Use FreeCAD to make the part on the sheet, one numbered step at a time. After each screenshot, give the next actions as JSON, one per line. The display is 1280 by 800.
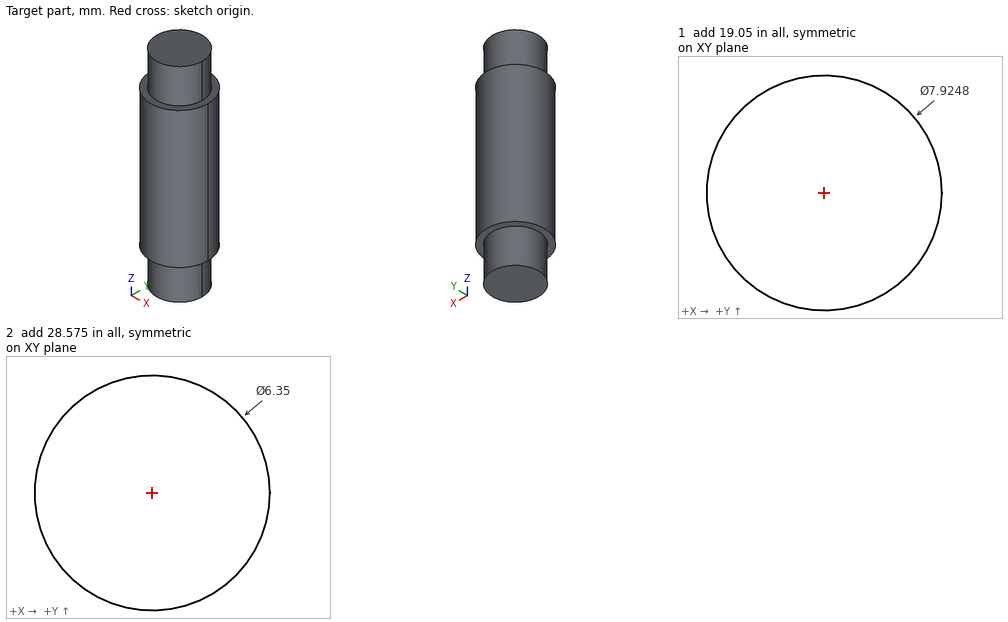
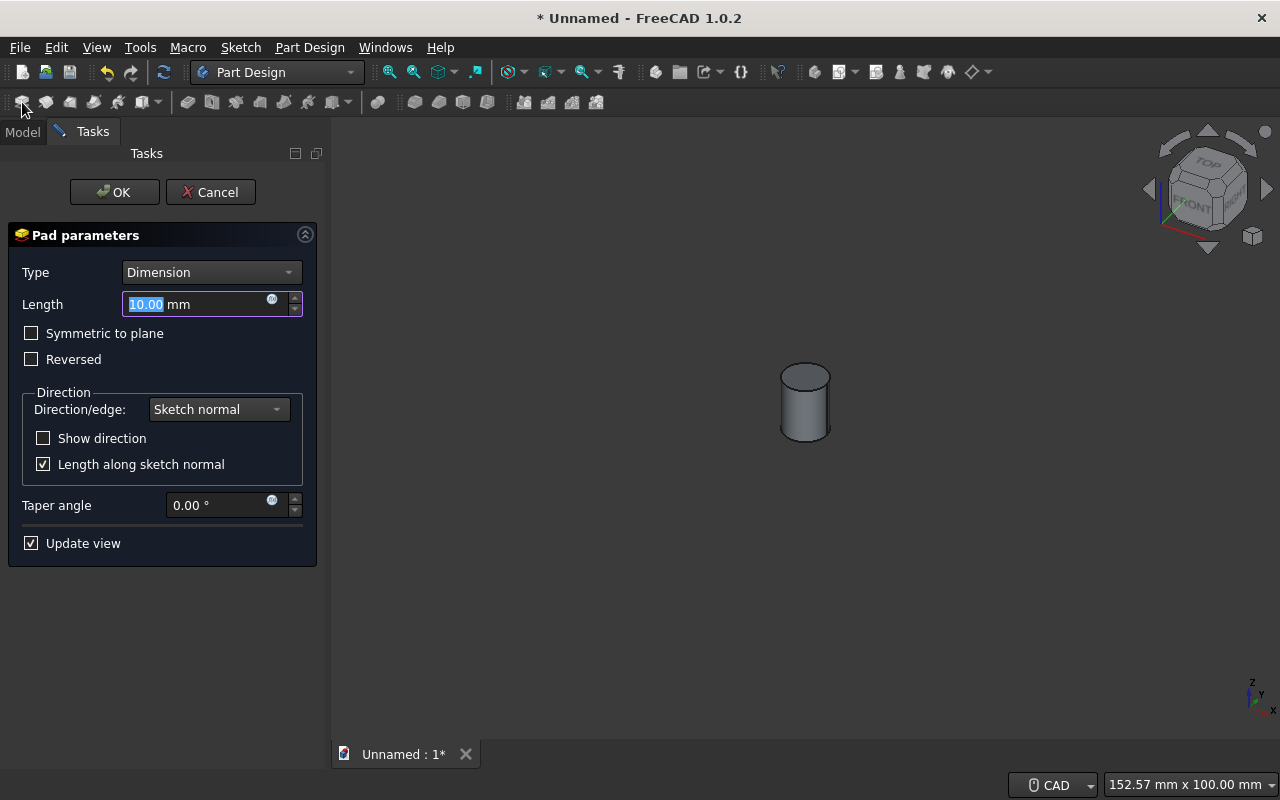
{"action": "type", "text": "19.05"}
{"action": "key", "text": "Tab"}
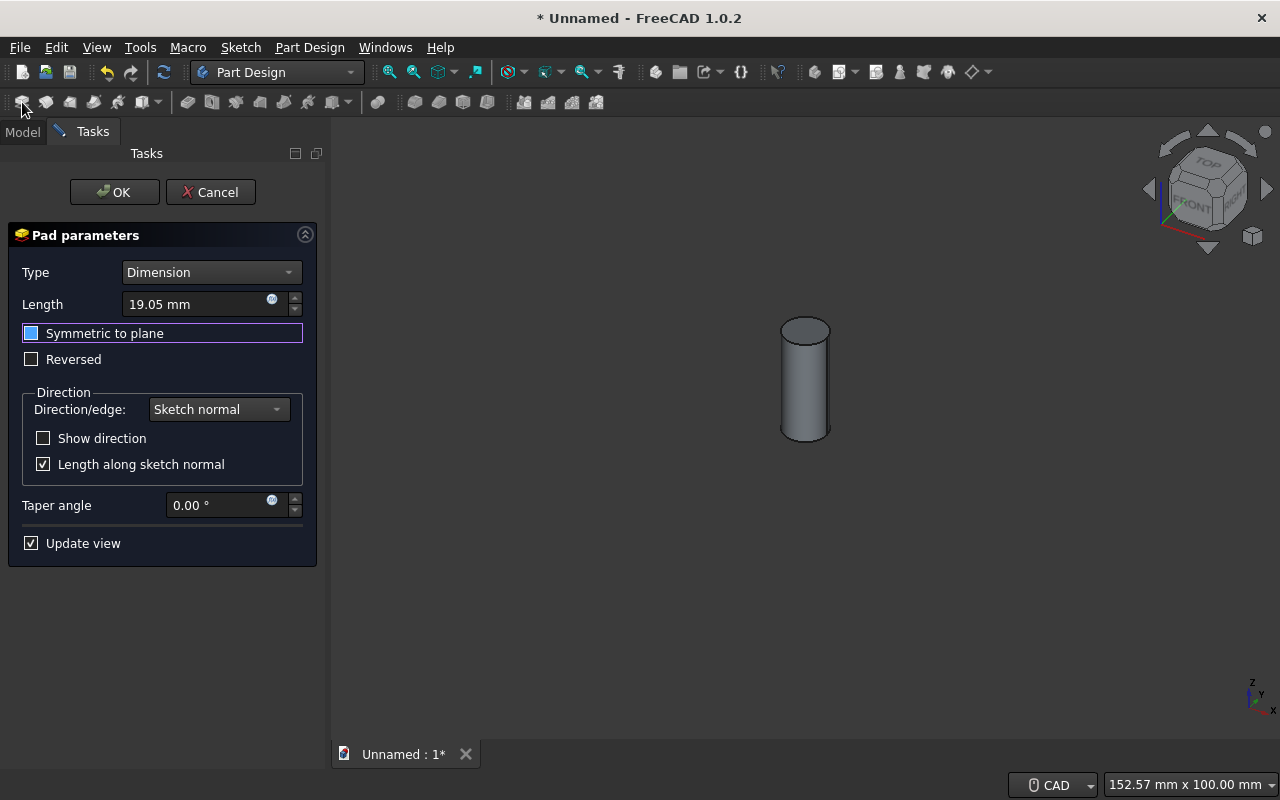
{"action": "left_click", "coordinate": [30, 333]}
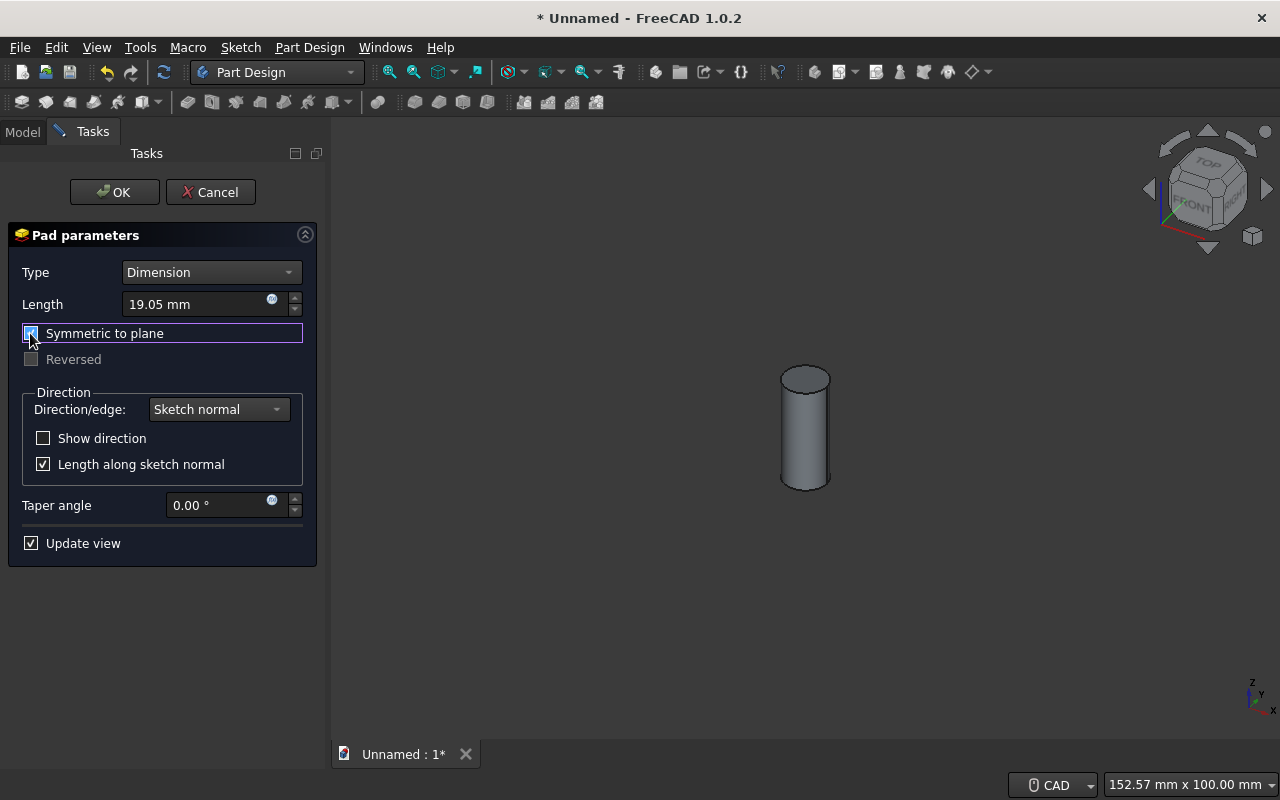
{"action": "left_click", "coordinate": [115, 192]}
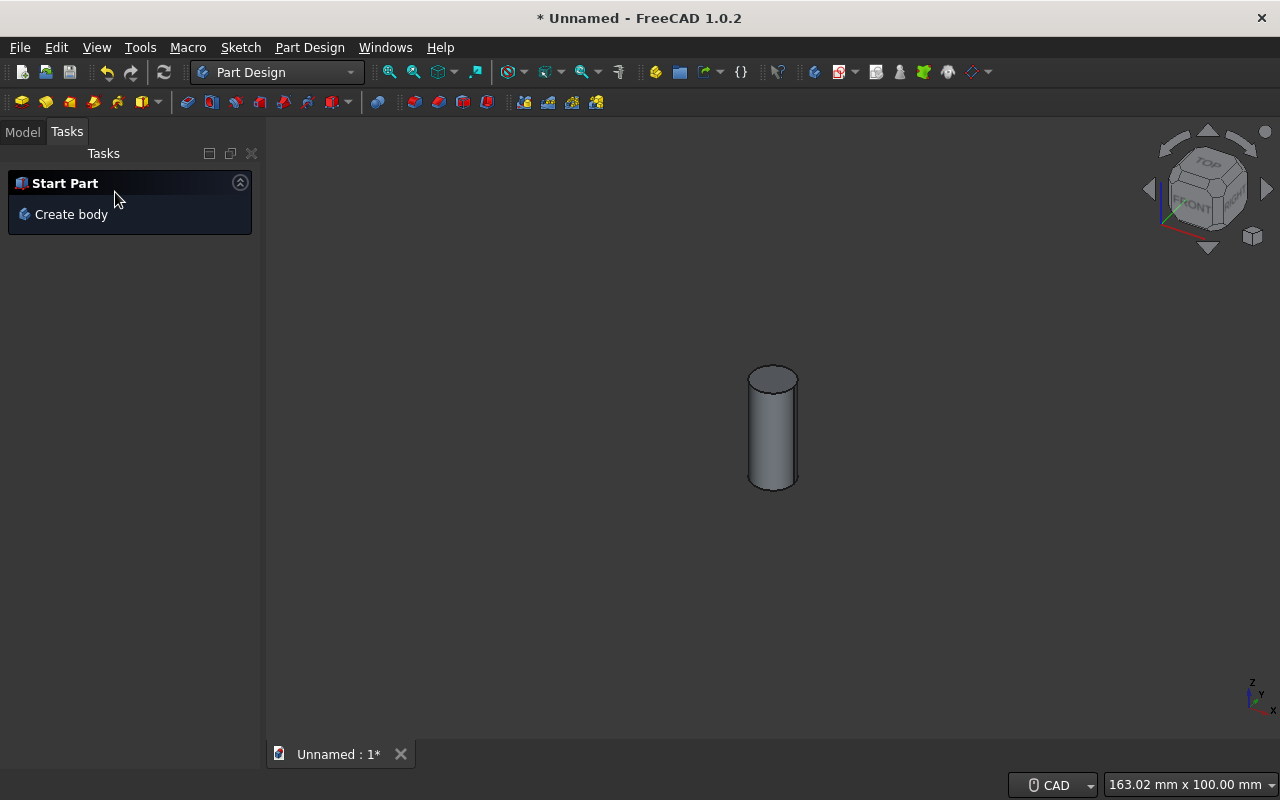
{"action": "key", "text": "v f"}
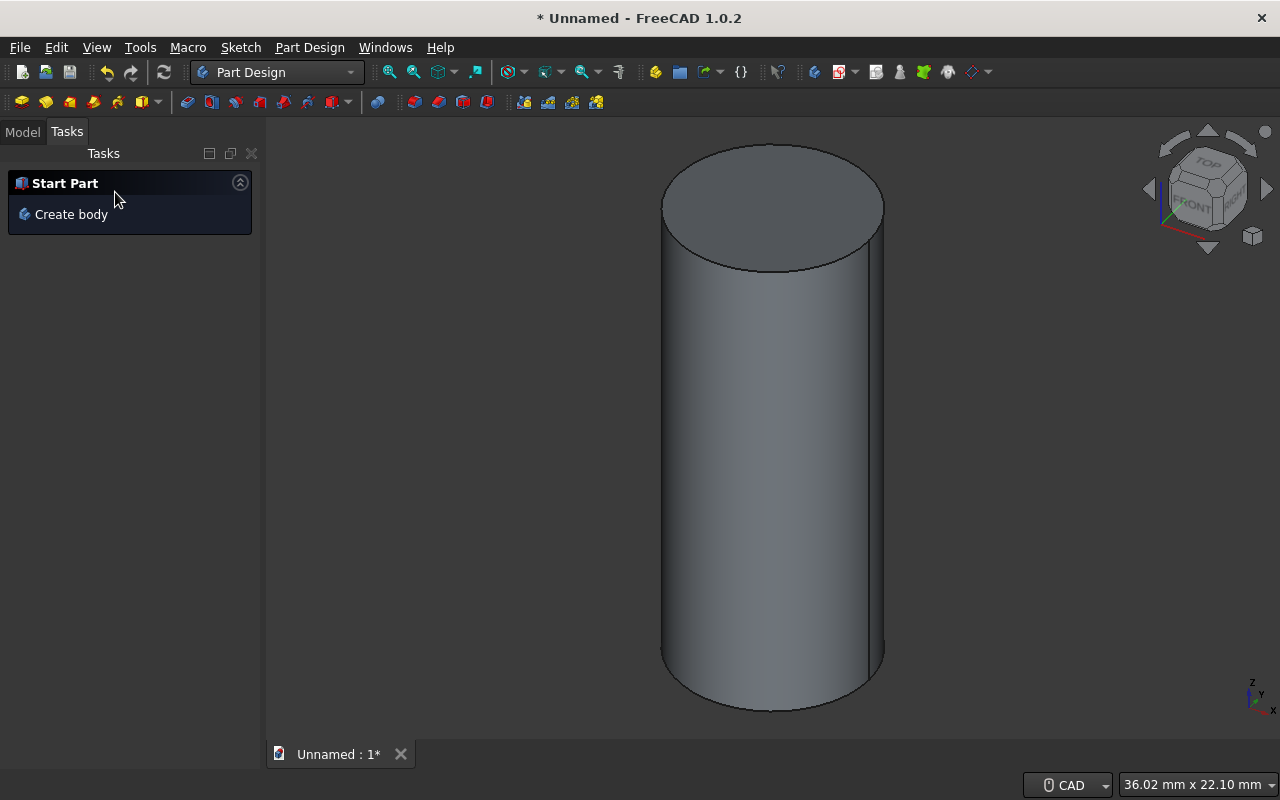
{"action": "left_click", "coordinate": [840, 72]}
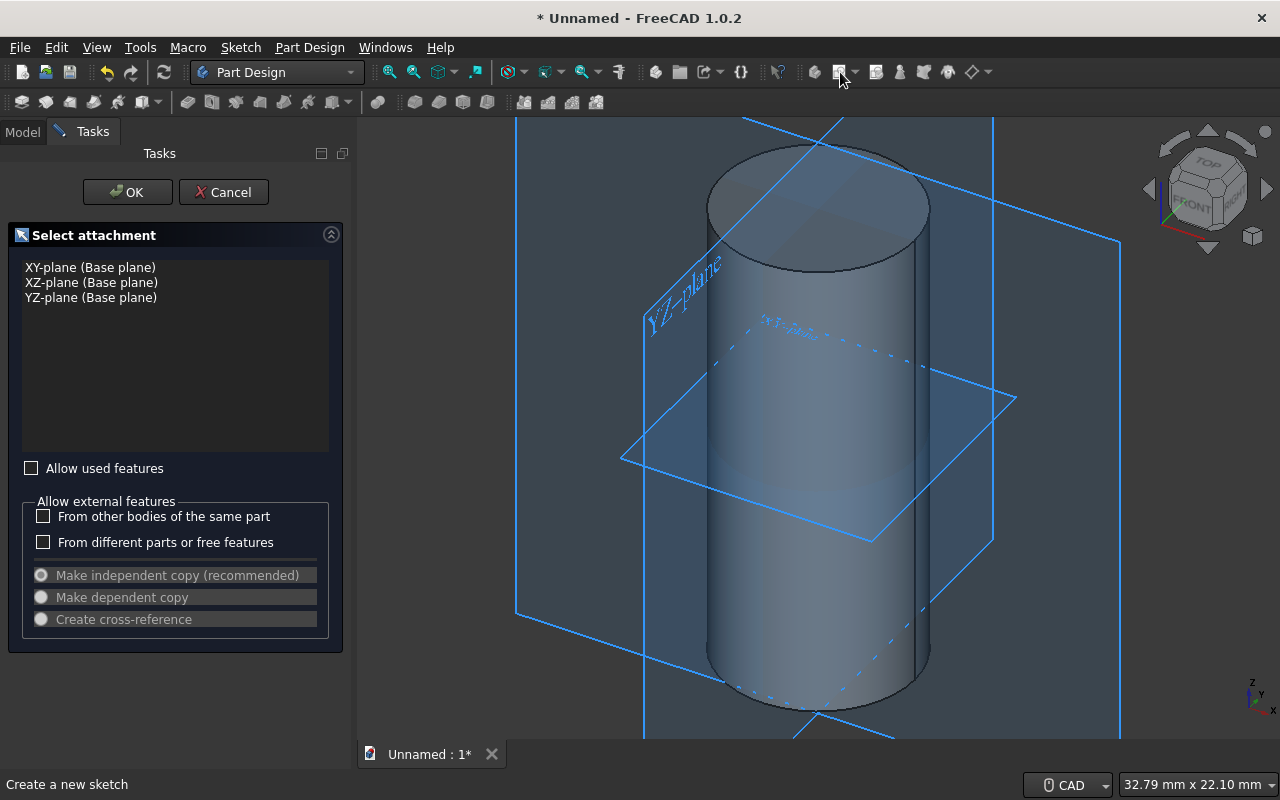
{"action": "left_click", "coordinate": [82, 268]}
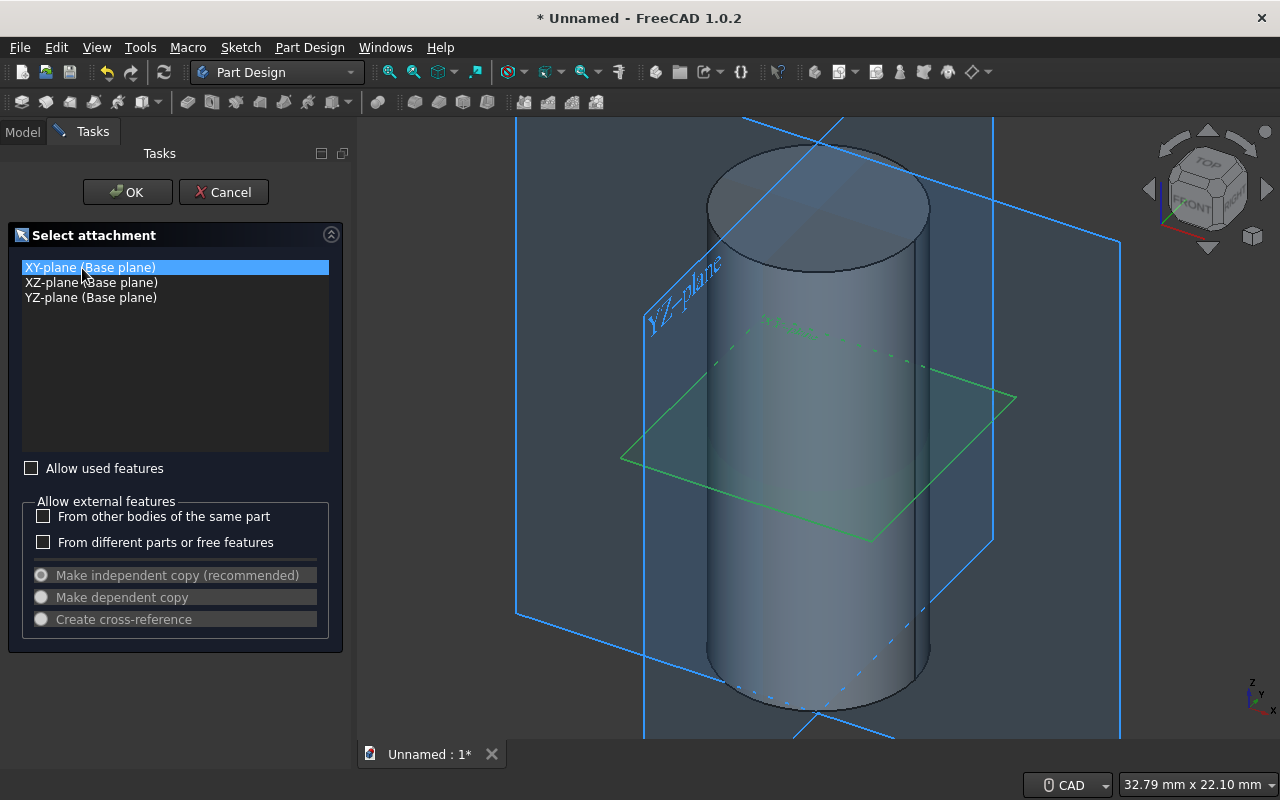
{"action": "left_click", "coordinate": [128, 192]}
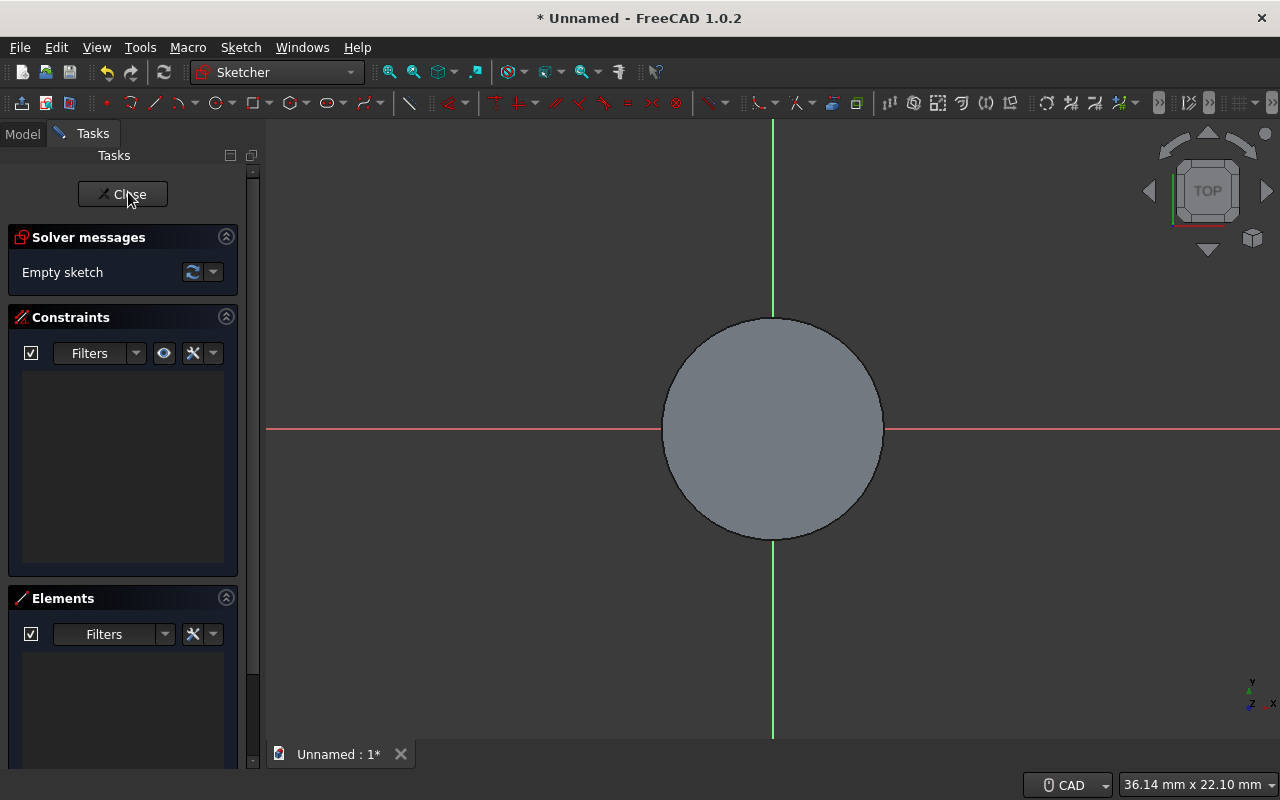
{"action": "left_click", "coordinate": [70, 104]}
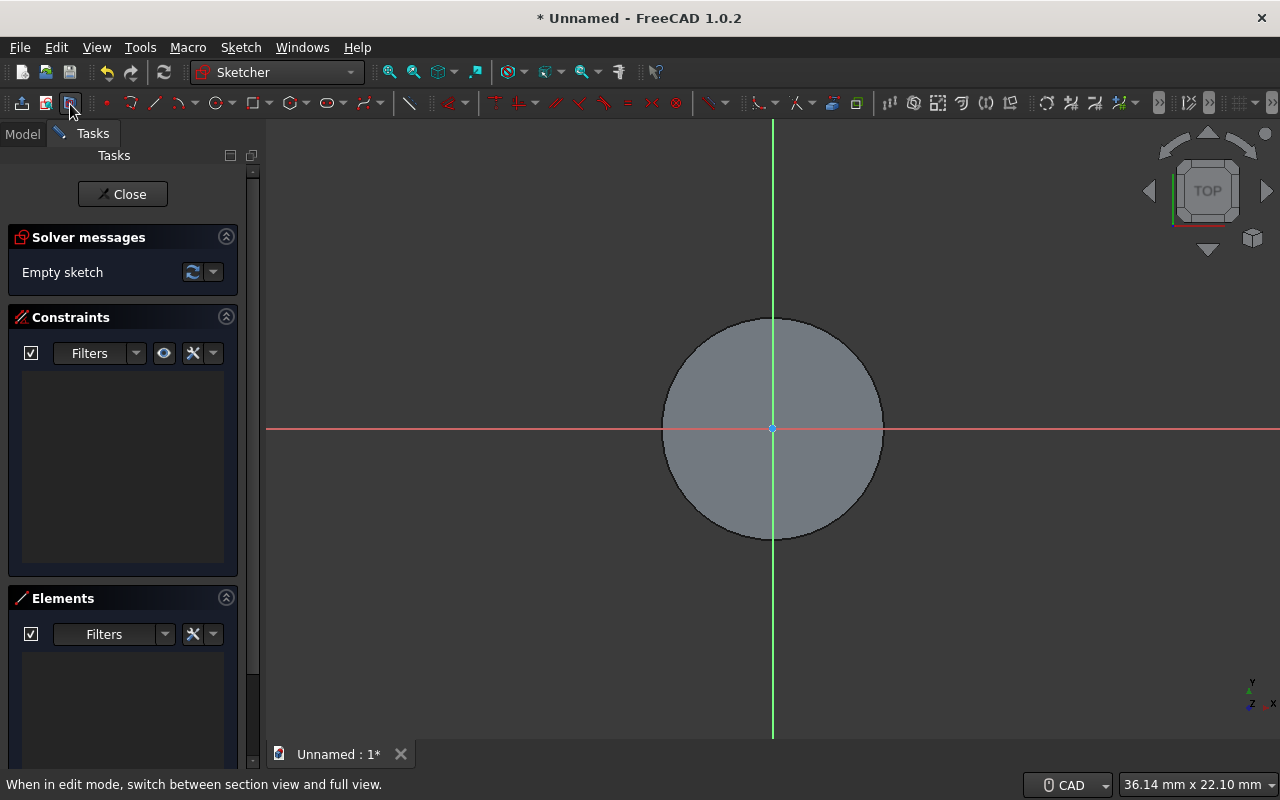
{"action": "scroll", "coordinate": [829, 429], "scroll_direction": "up", "scroll_amount": 4}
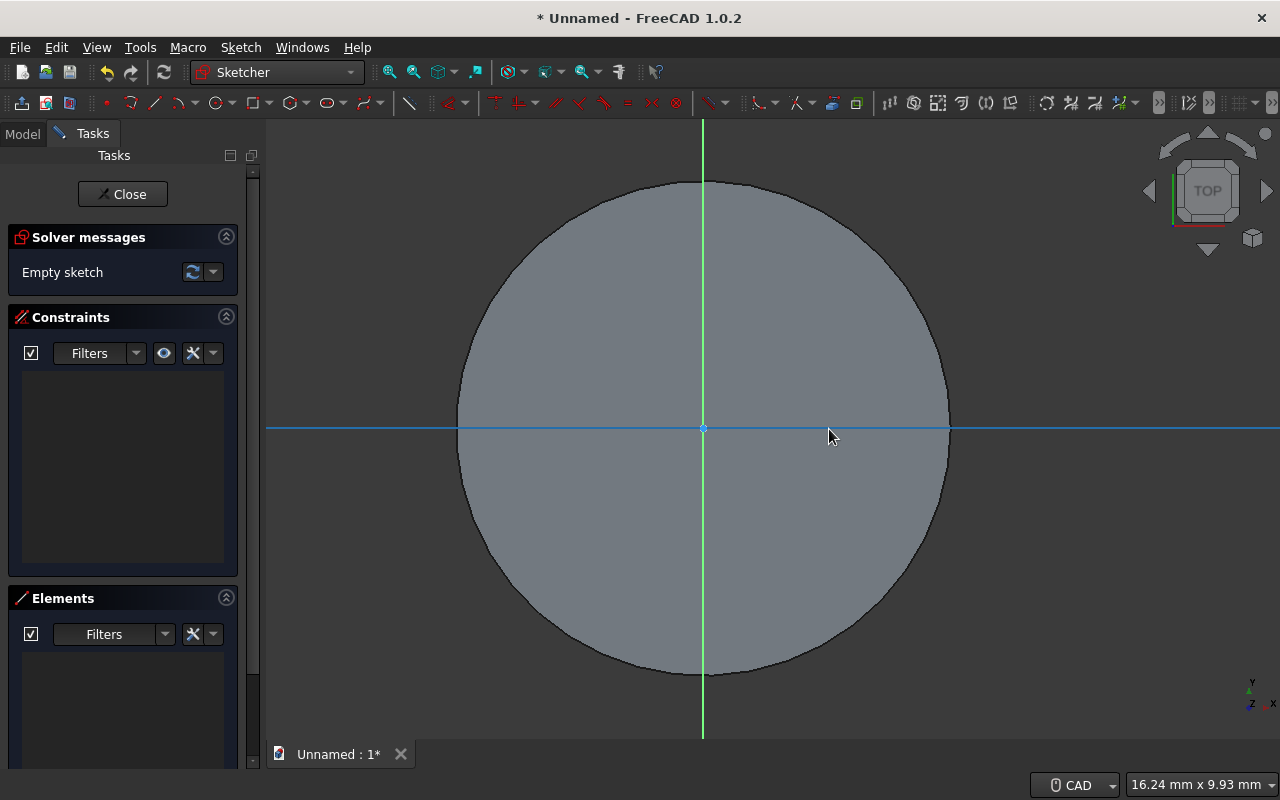
{"action": "left_click", "coordinate": [216, 104]}